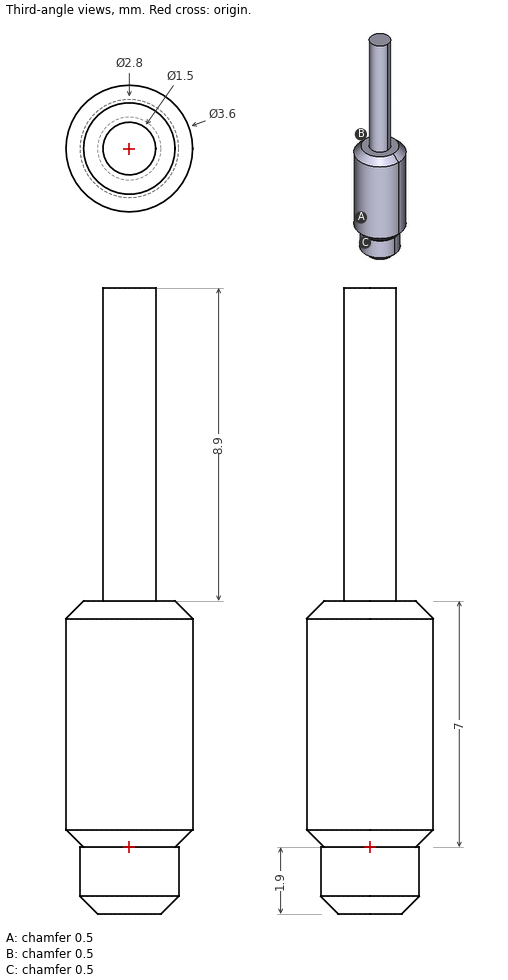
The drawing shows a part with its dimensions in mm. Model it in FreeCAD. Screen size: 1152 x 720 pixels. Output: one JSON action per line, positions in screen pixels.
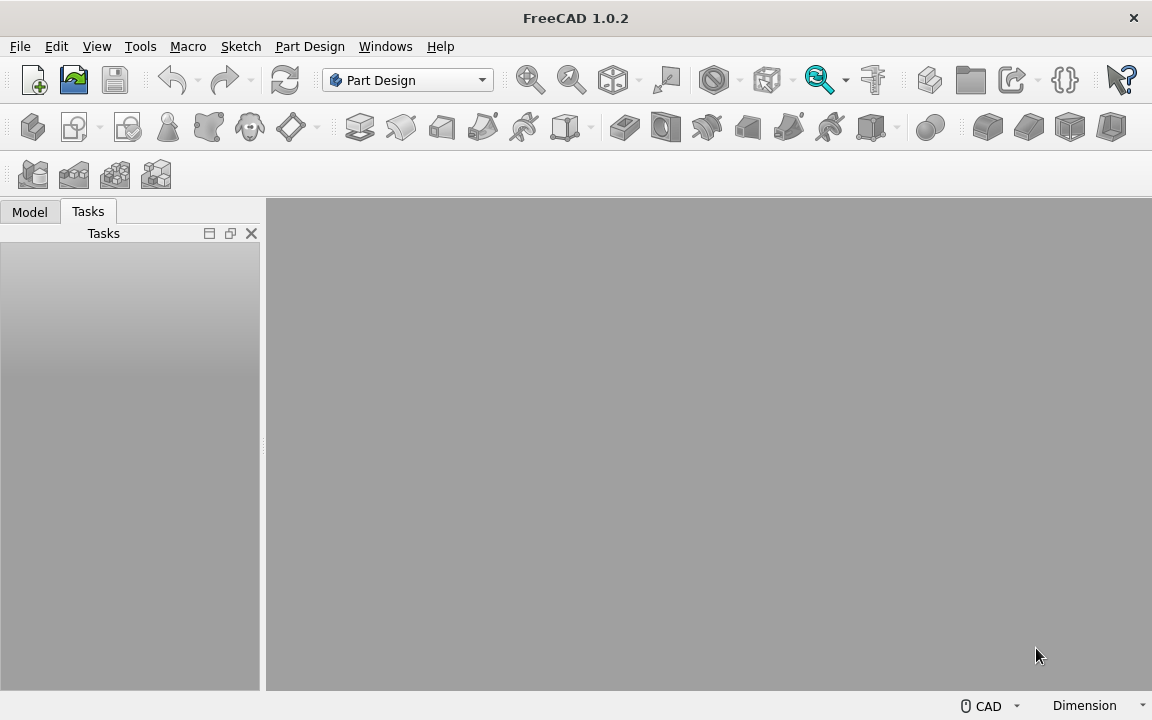
{"action": "left_click", "coordinate": [33, 80]}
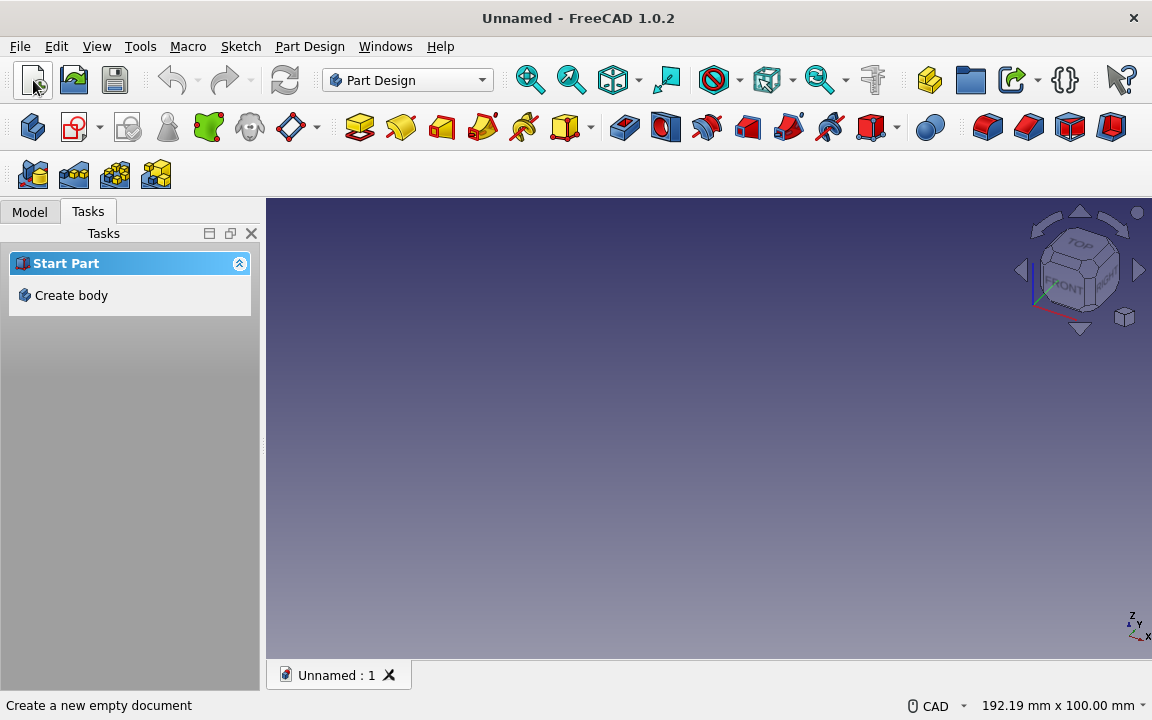
{"action": "left_click", "coordinate": [74, 128]}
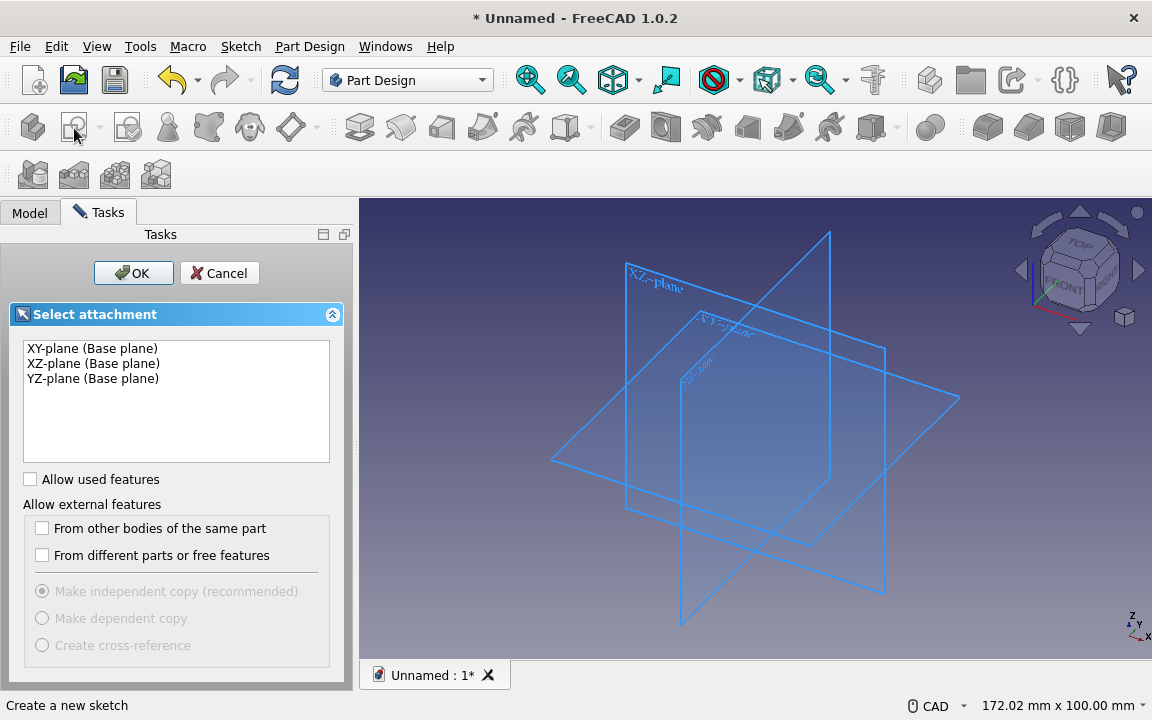
{"action": "left_click", "coordinate": [84, 348]}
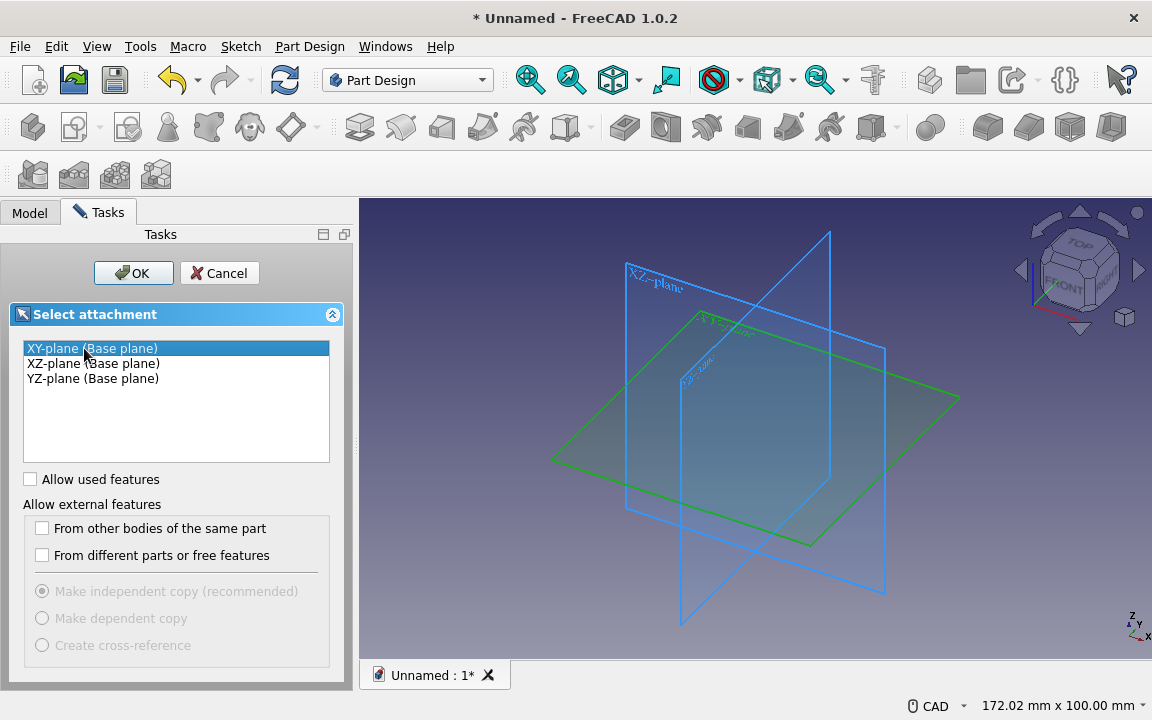
{"action": "left_click", "coordinate": [134, 273]}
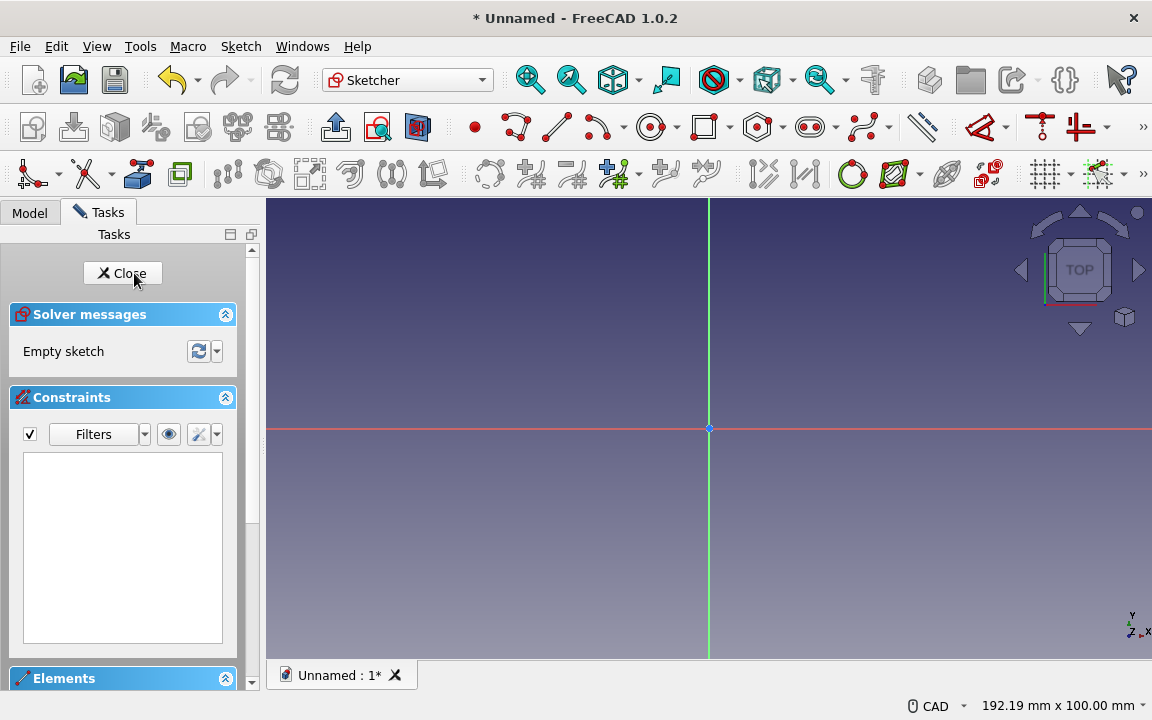
{"action": "scroll", "coordinate": [713, 428], "scroll_direction": "up", "scroll_amount": 14}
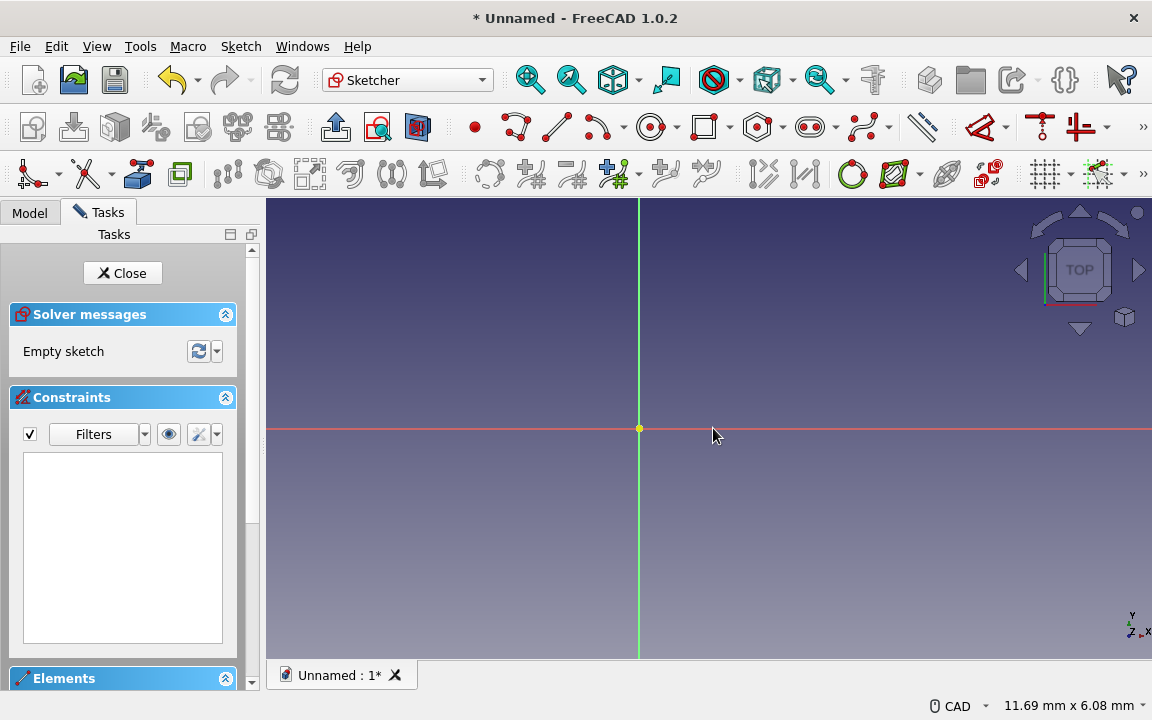
{"action": "key", "text": "g c"}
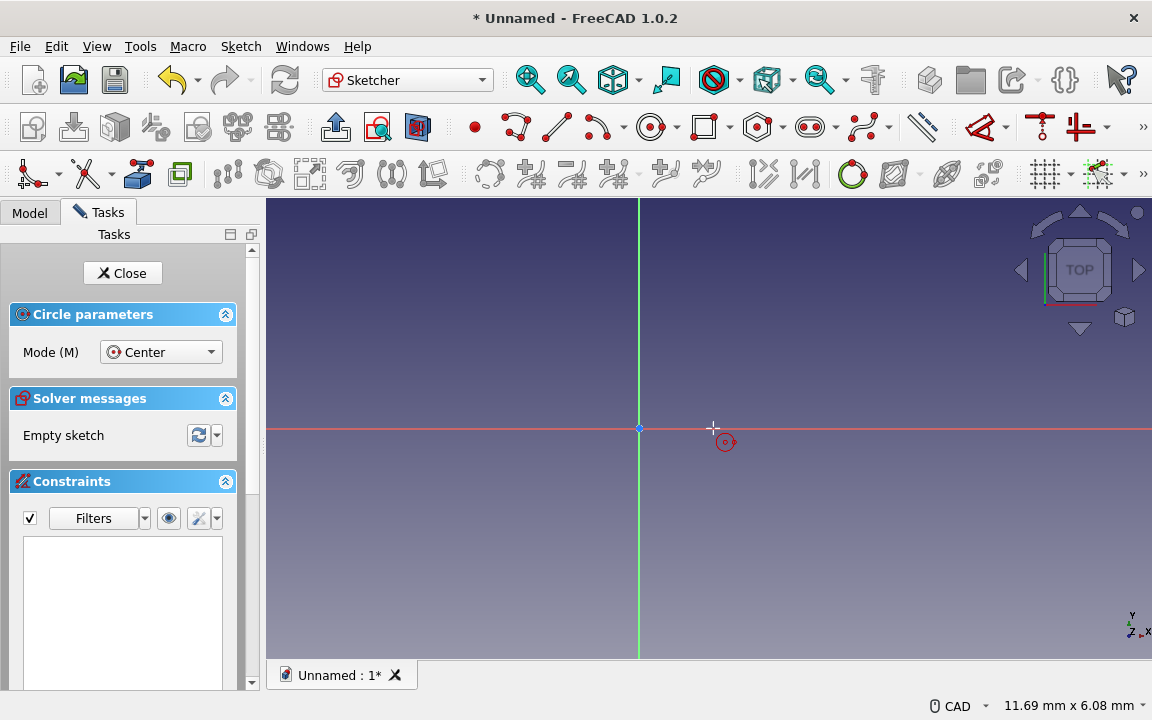
{"action": "left_click", "coordinate": [639, 428]}
{"action": "mouse_move", "coordinate": [736, 332]}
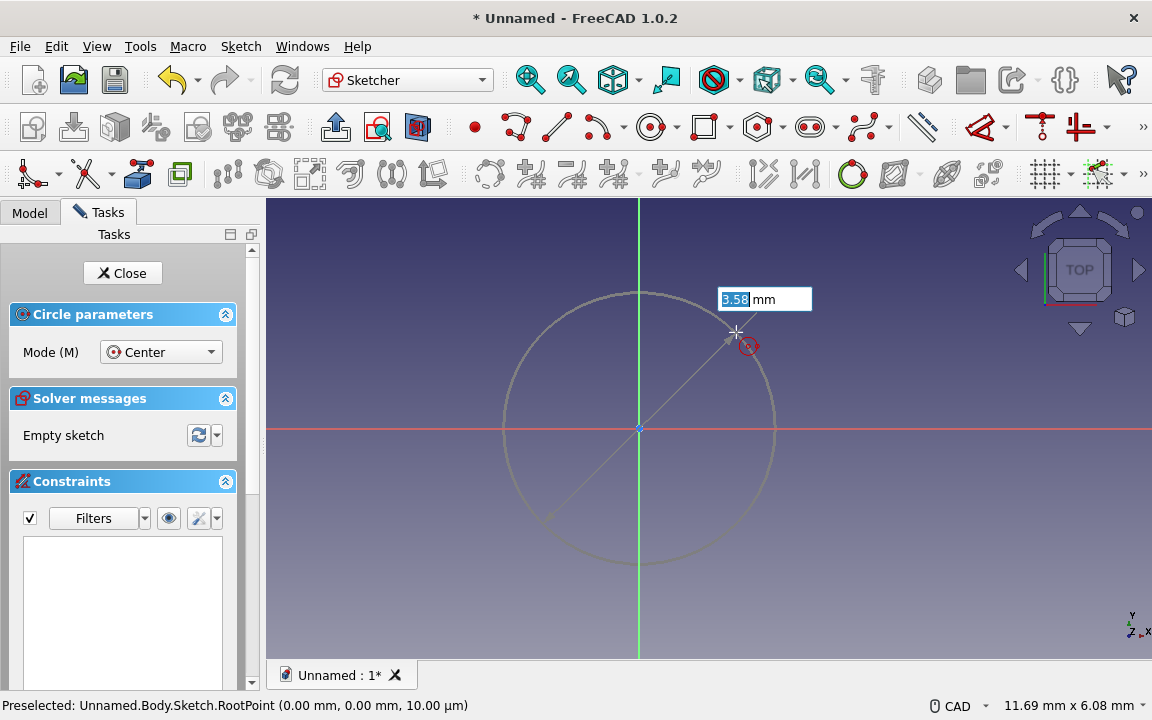
{"action": "type", "text": "3.6"}
{"action": "key", "text": "Return"}
{"action": "key", "text": "Escape"}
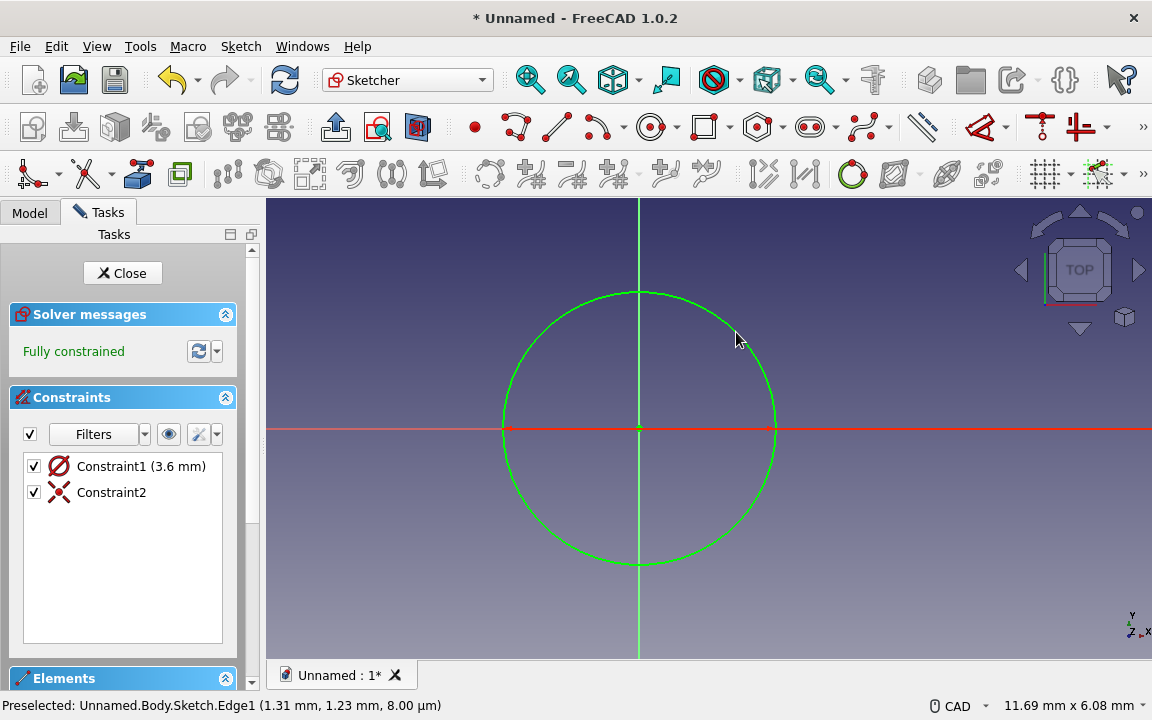
{"action": "left_click", "coordinate": [123, 273]}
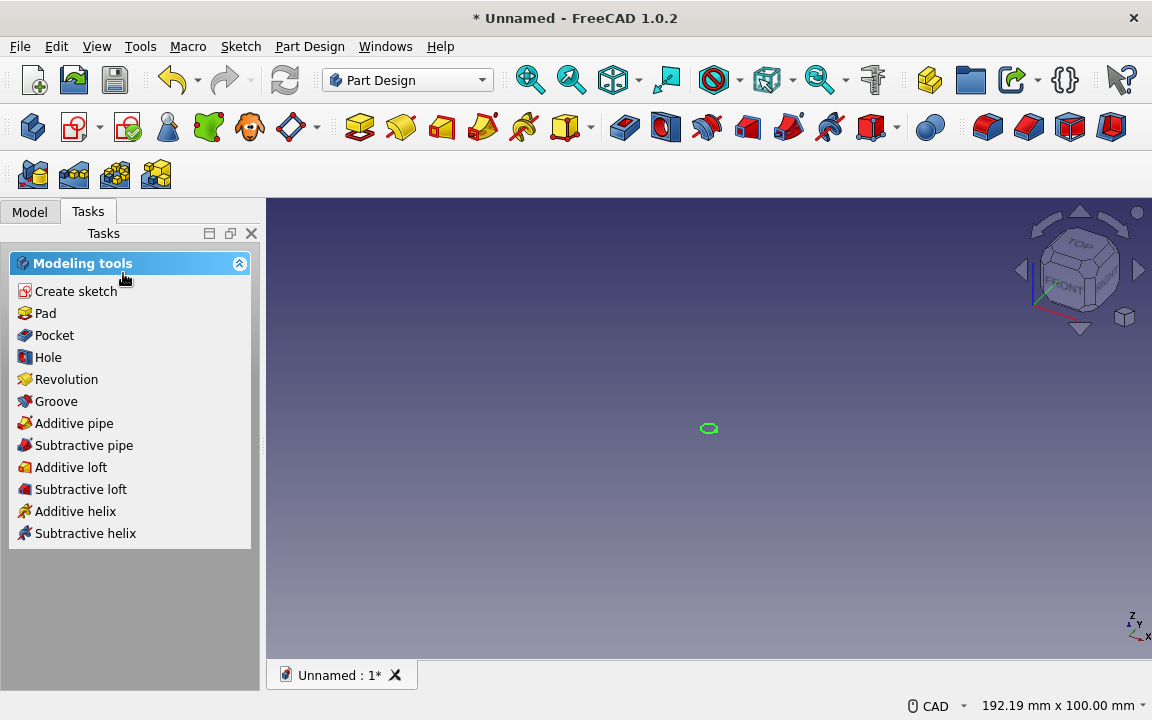
{"action": "left_click", "coordinate": [360, 128]}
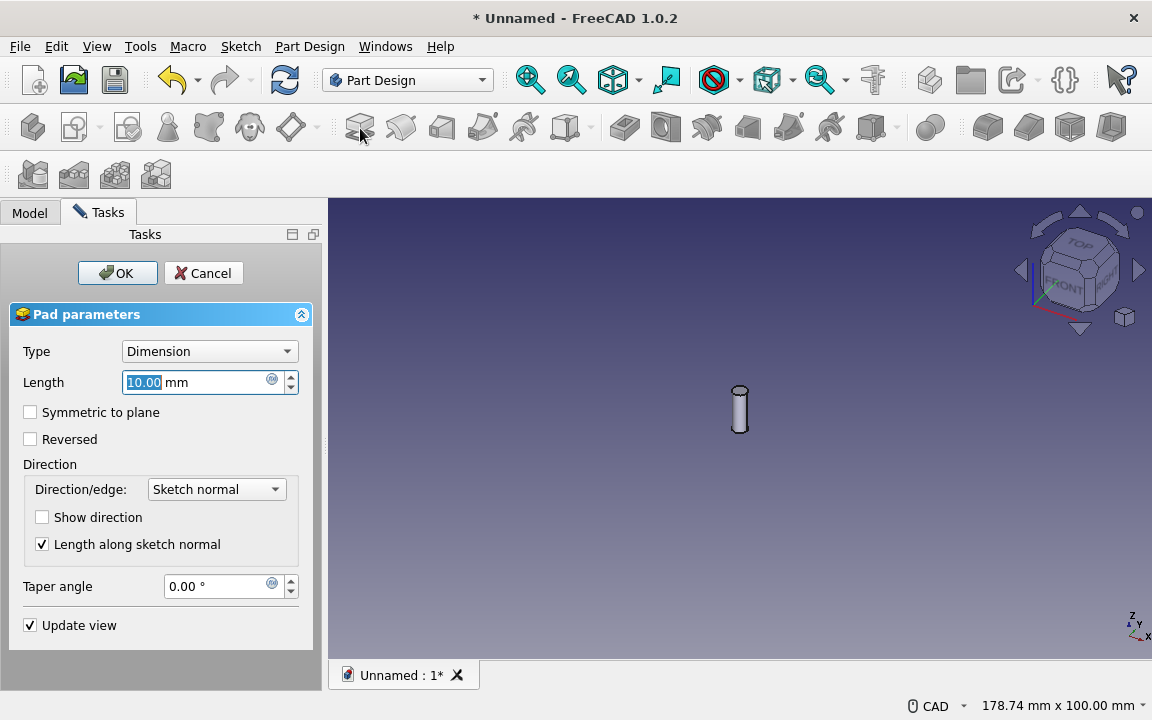
{"action": "type", "text": "7"}
{"action": "key", "text": "Tab"}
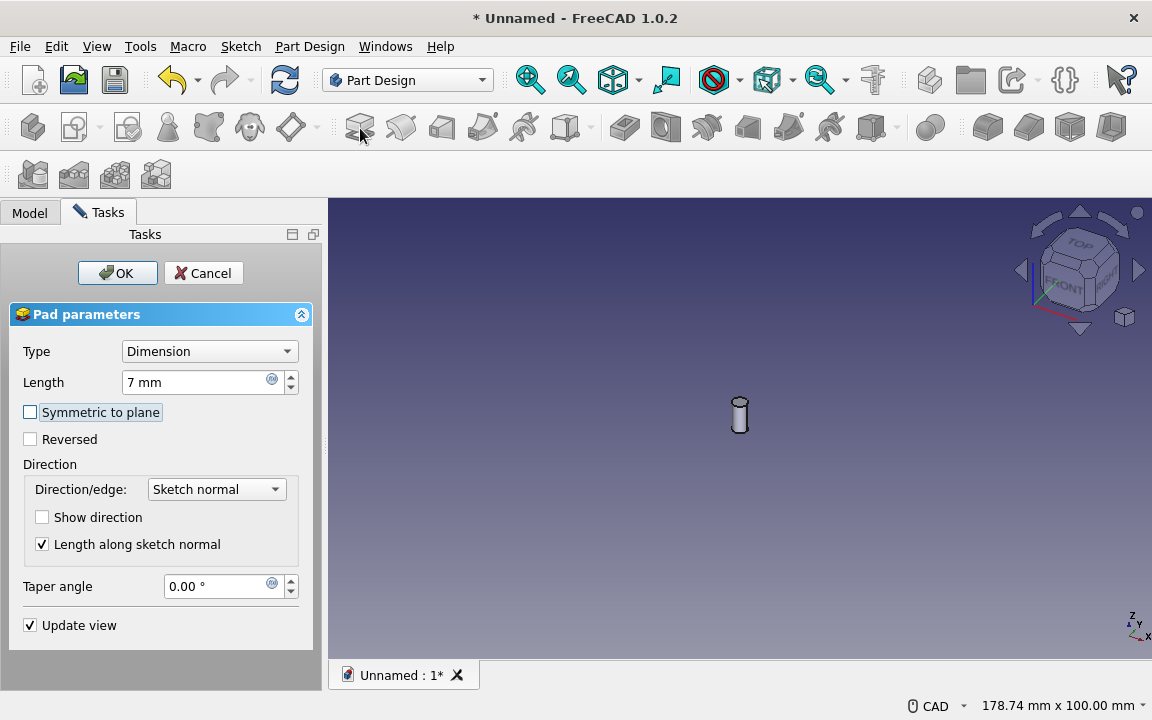
{"action": "left_click", "coordinate": [118, 273]}